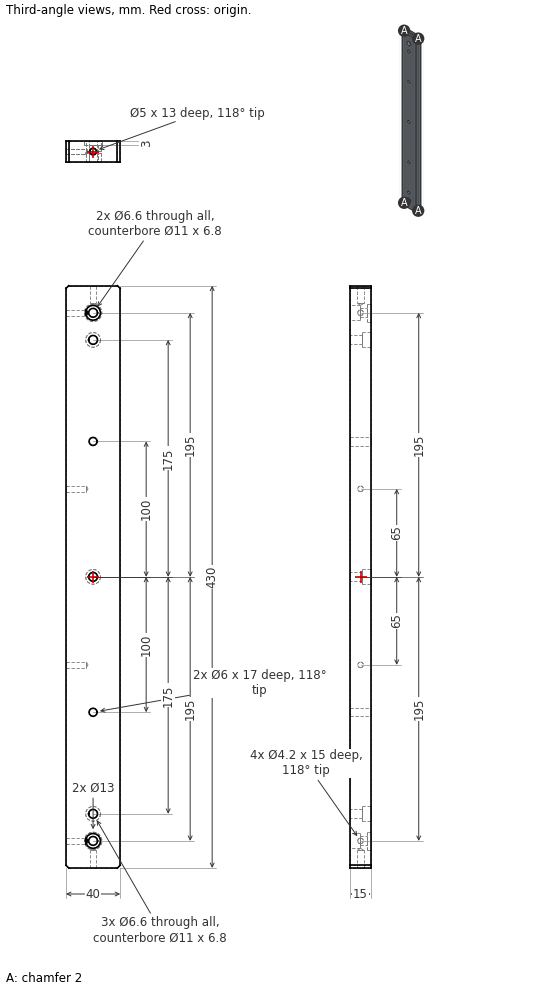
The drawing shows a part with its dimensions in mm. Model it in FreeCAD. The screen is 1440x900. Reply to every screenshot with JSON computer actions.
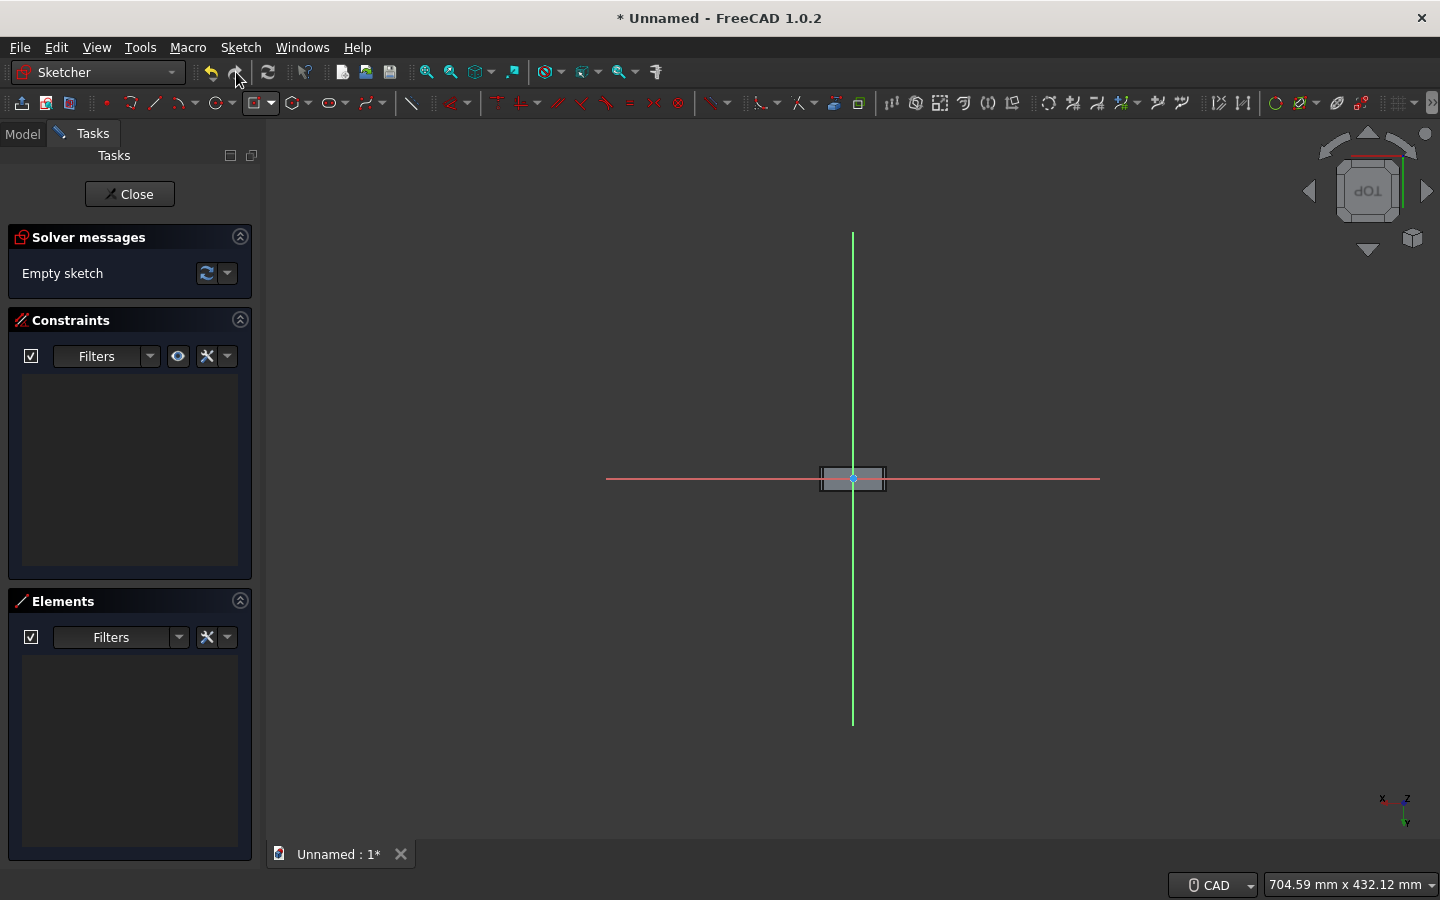
{"action": "scroll", "coordinate": [857, 479], "scroll_direction": "up", "scroll_amount": 15}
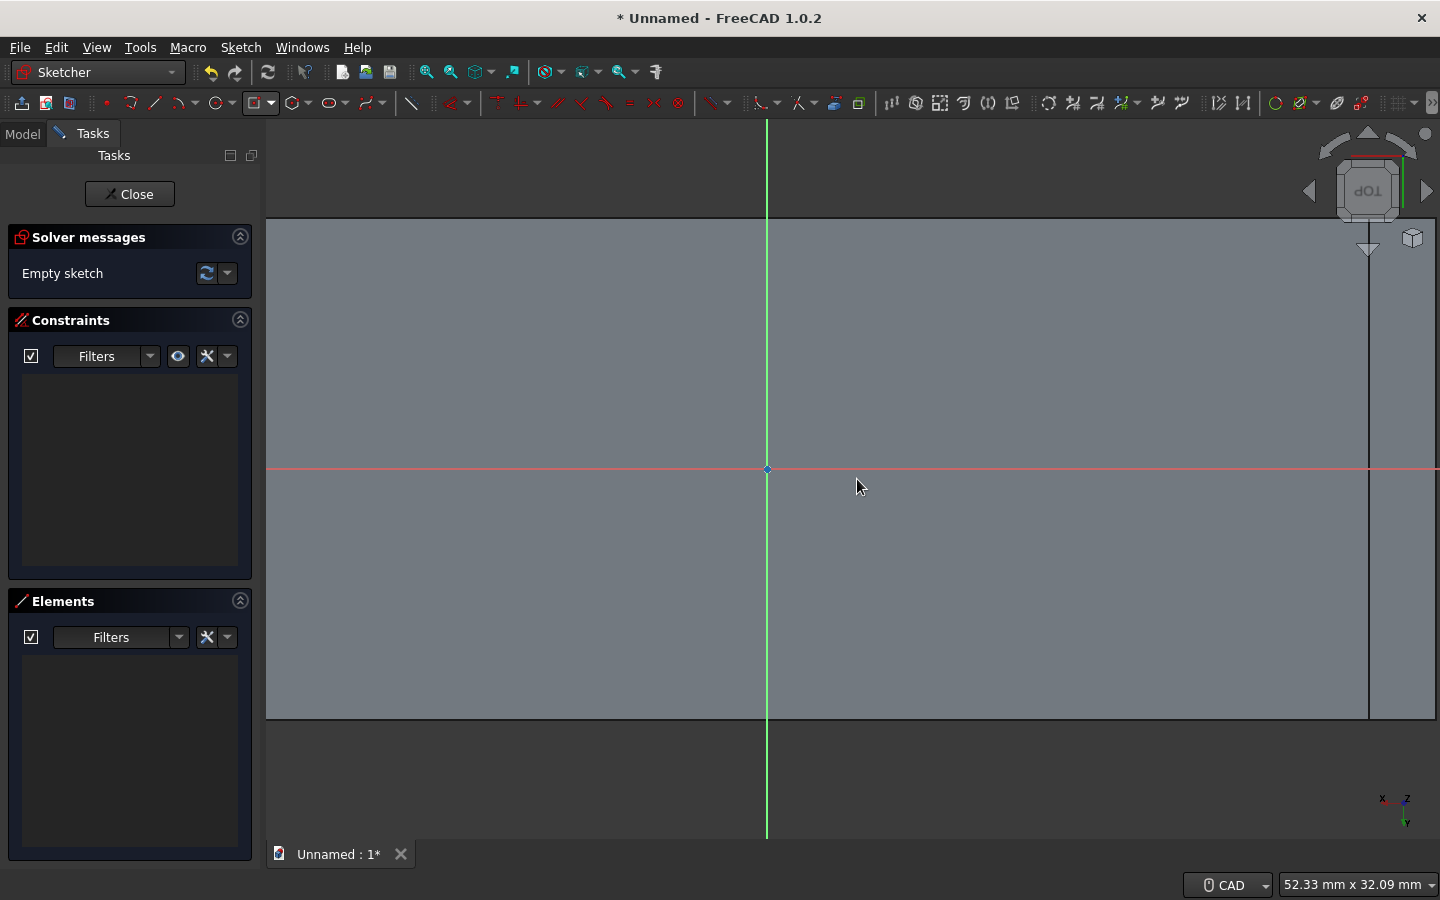
{"action": "scroll", "coordinate": [757, 464], "scroll_direction": "up", "scroll_amount": 5}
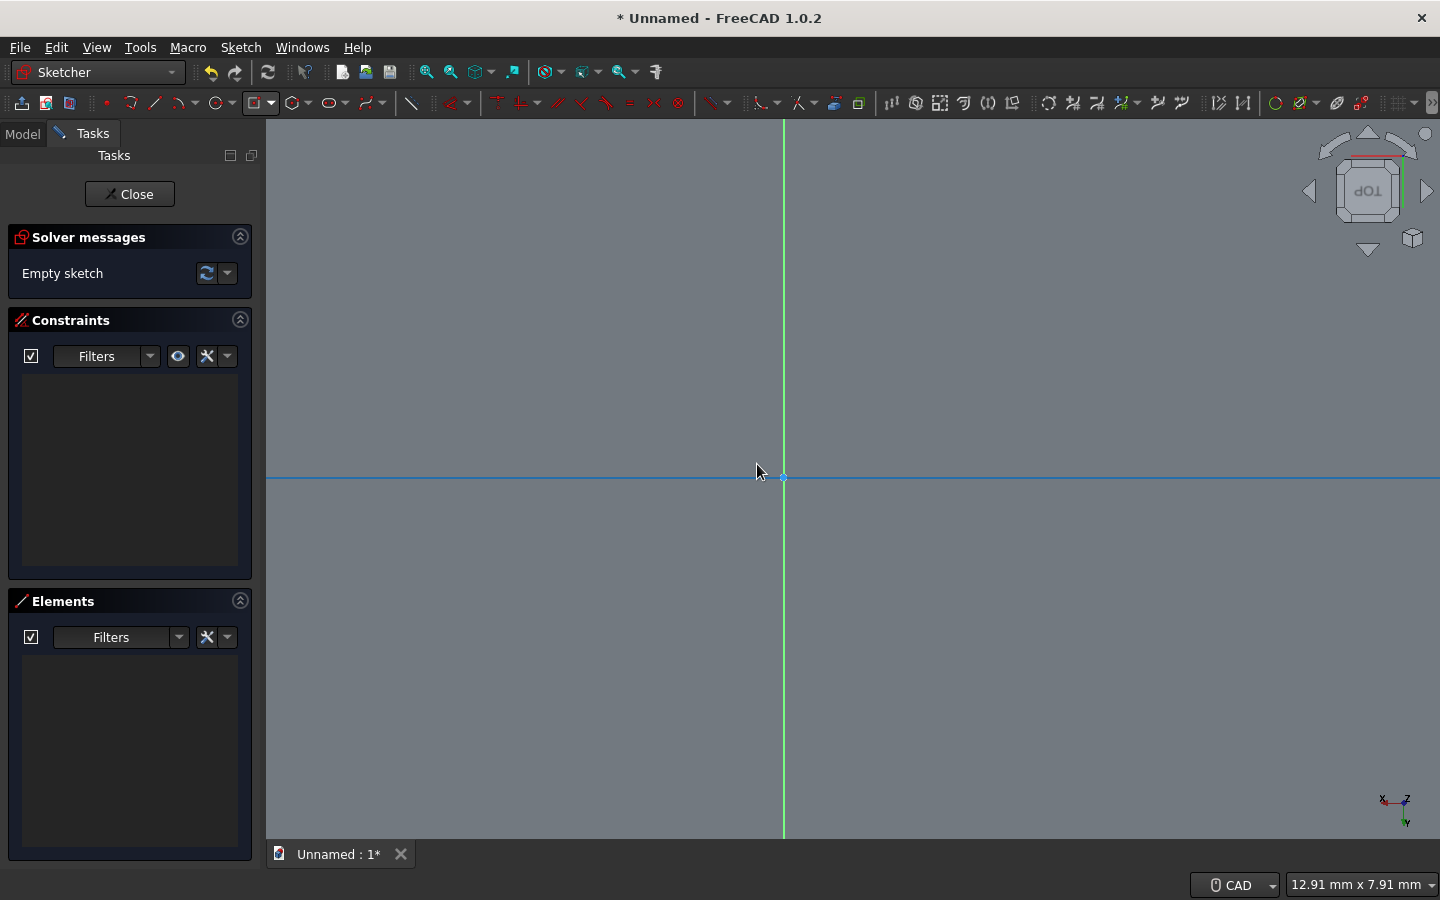
{"action": "key", "text": "g c"}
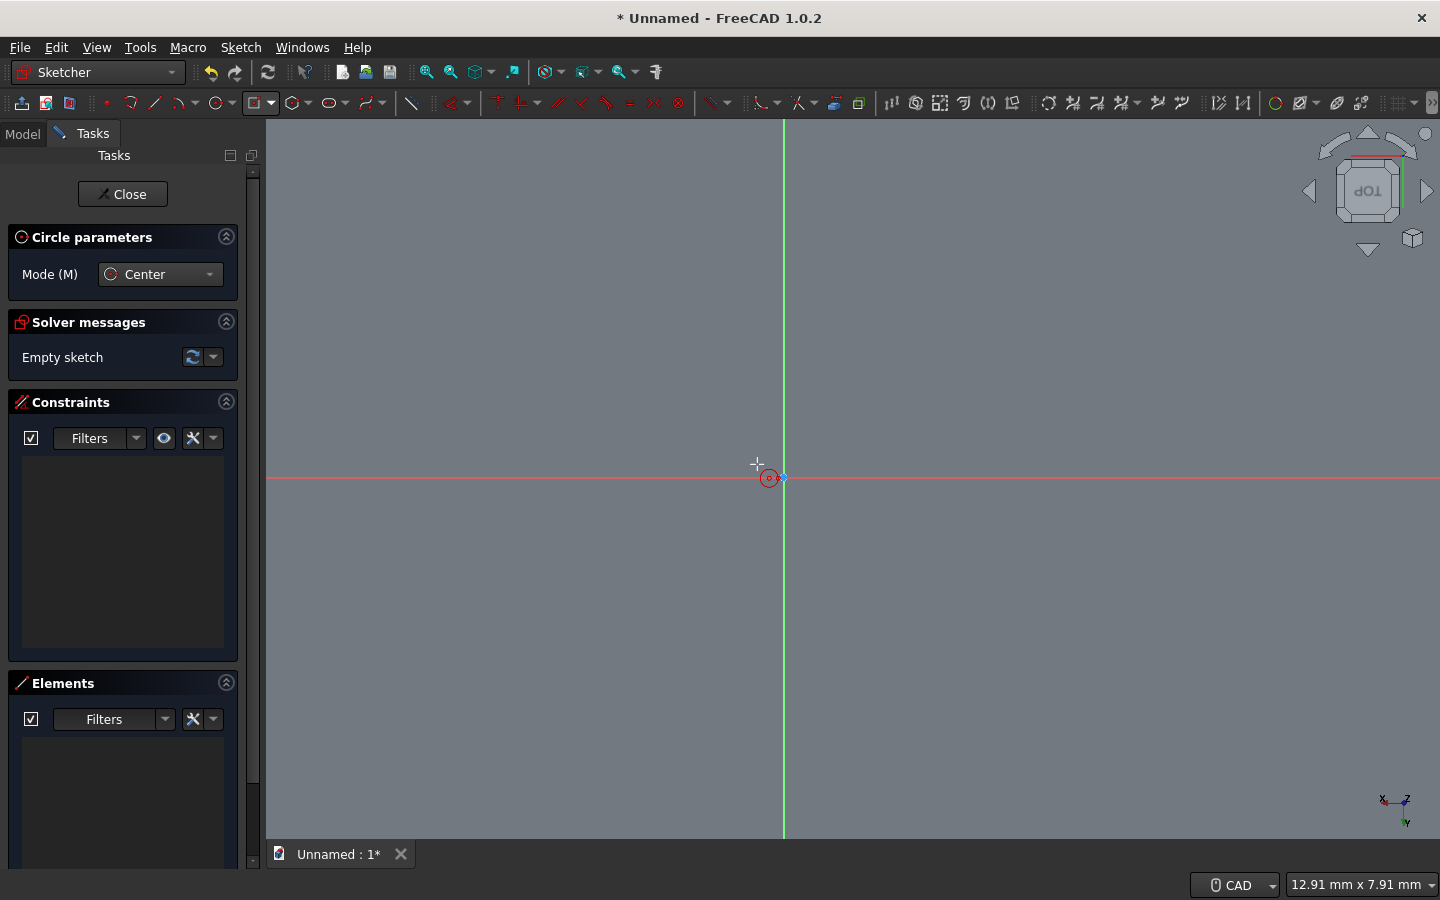
{"action": "left_click", "coordinate": [784, 478]}
{"action": "left_click", "coordinate": [944, 317]}
{"action": "key", "text": "Escape"}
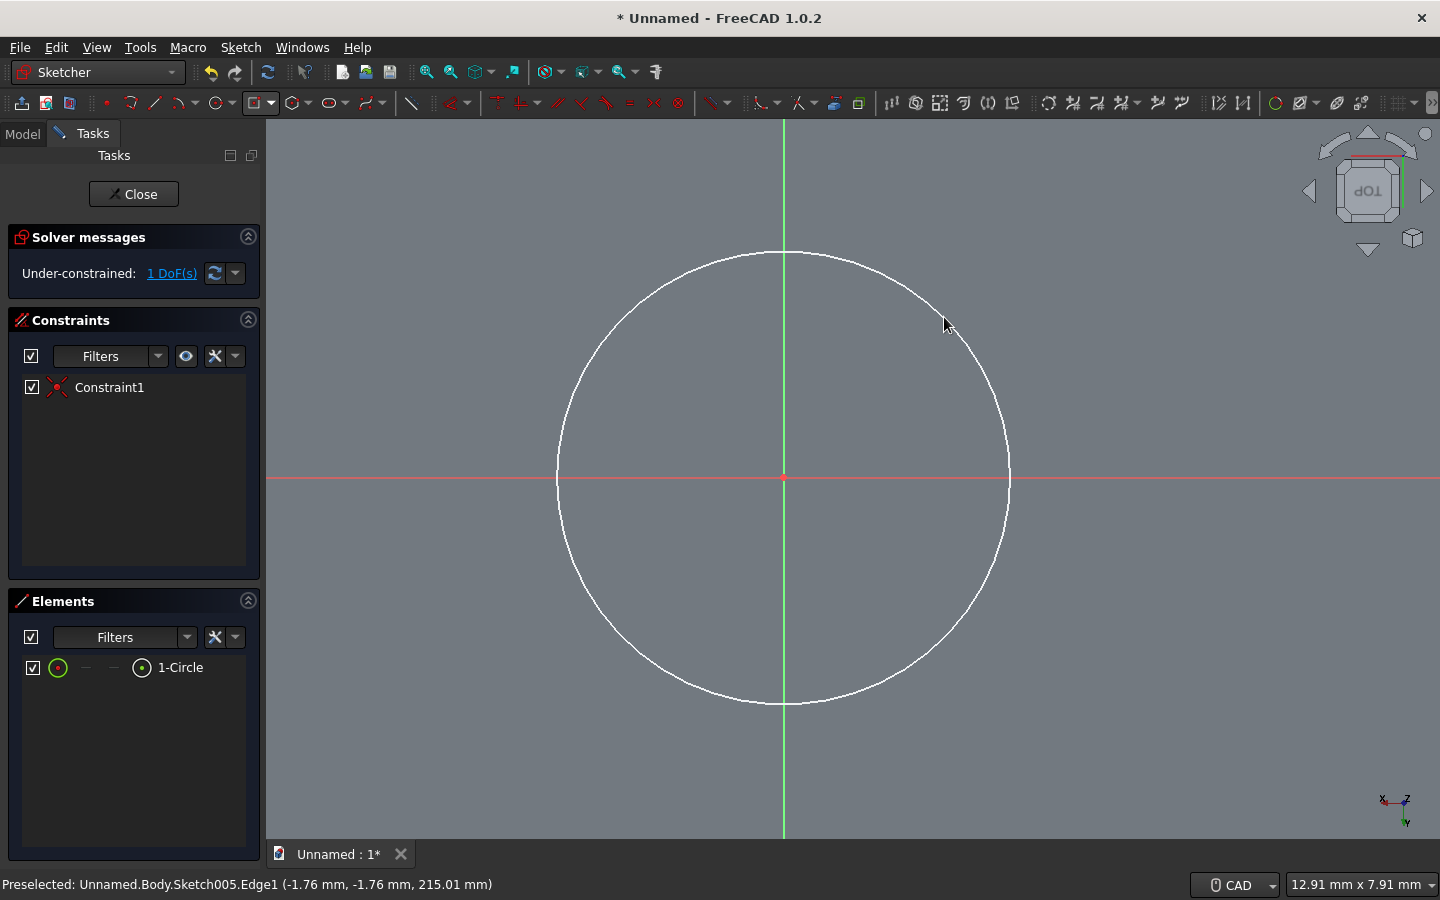
{"action": "key", "text": "d"}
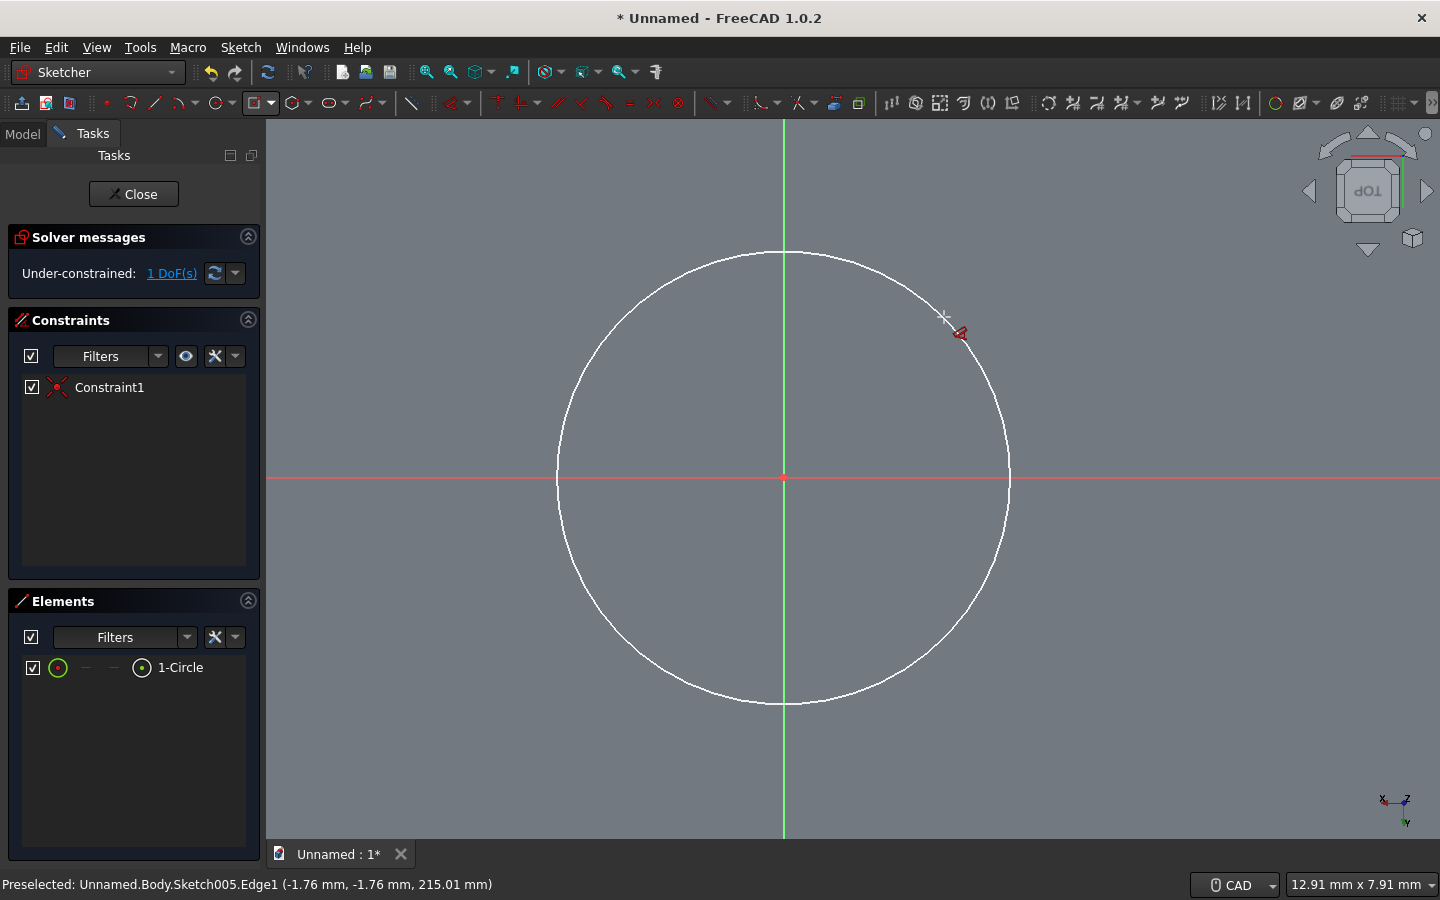
{"action": "left_click", "coordinate": [943, 317]}
{"action": "left_click", "coordinate": [966, 294]}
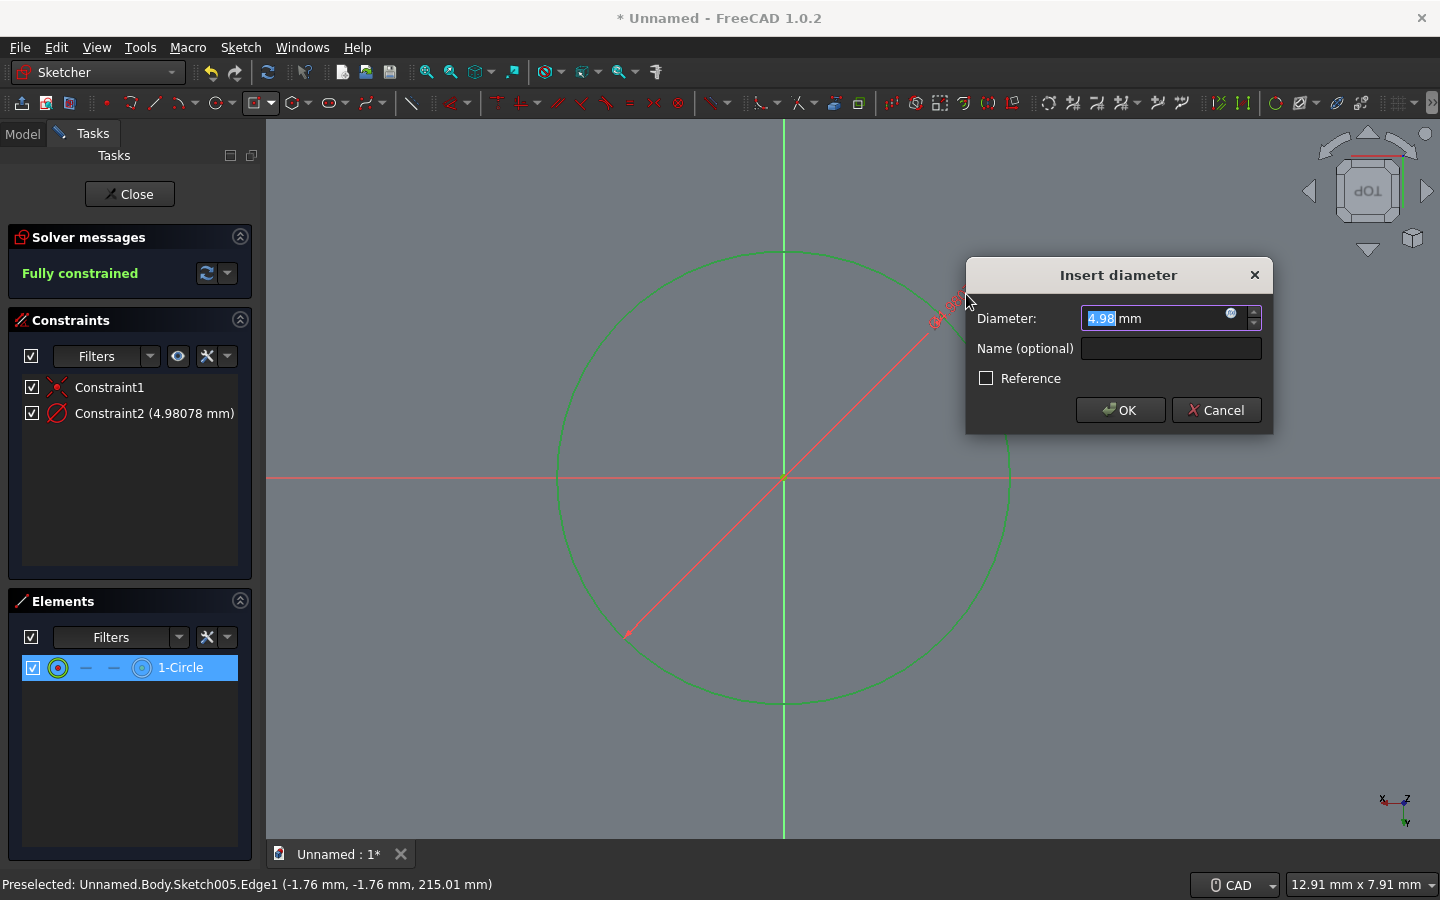
{"action": "type", "text": "5"}
{"action": "key", "text": "Return"}
{"action": "key", "text": "Escape"}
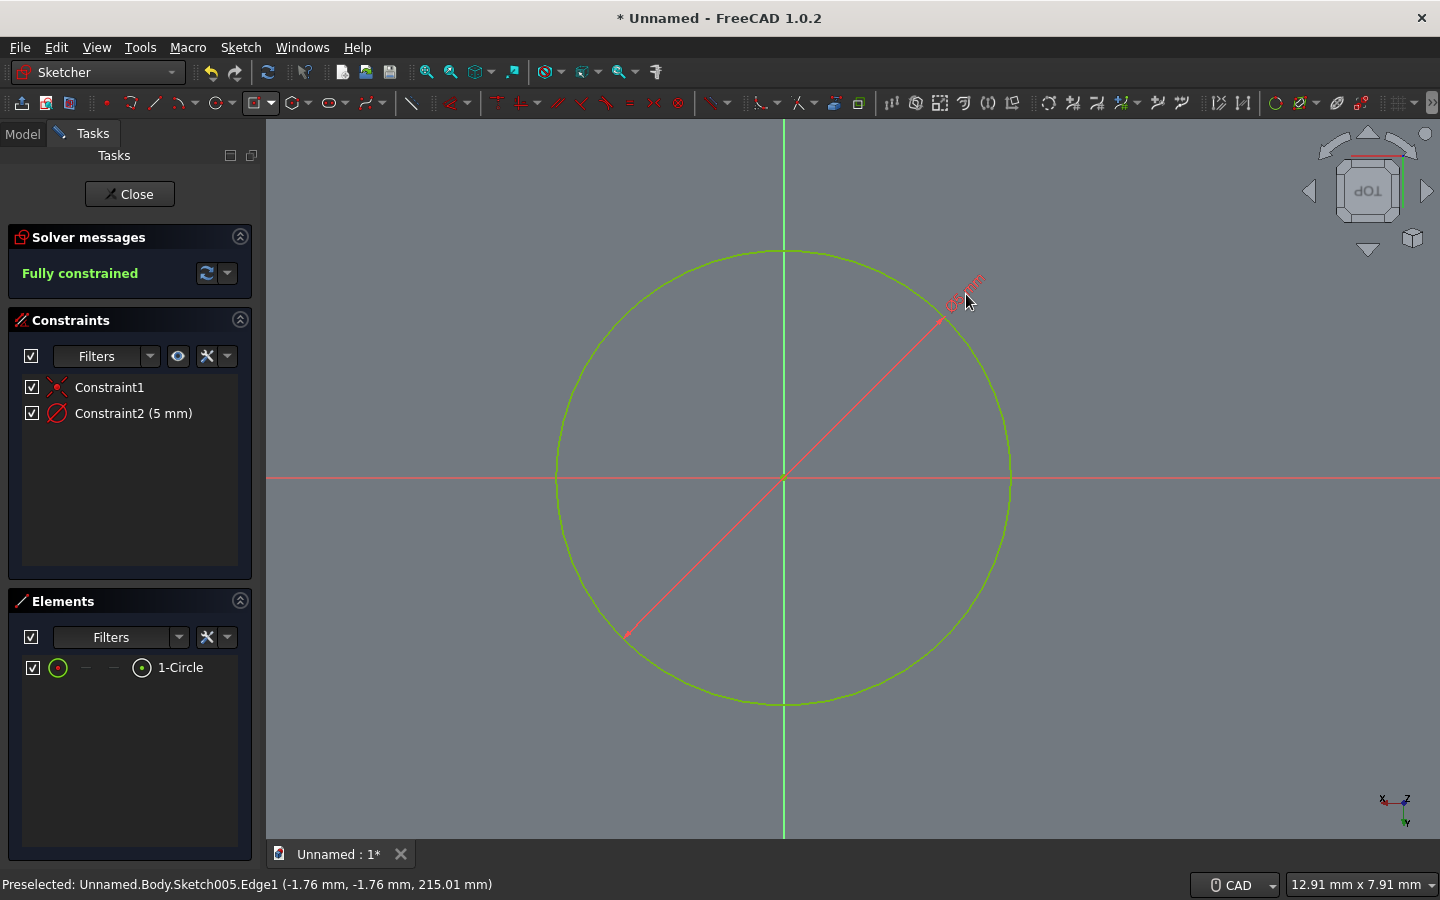
{"action": "left_click", "coordinate": [130, 194]}